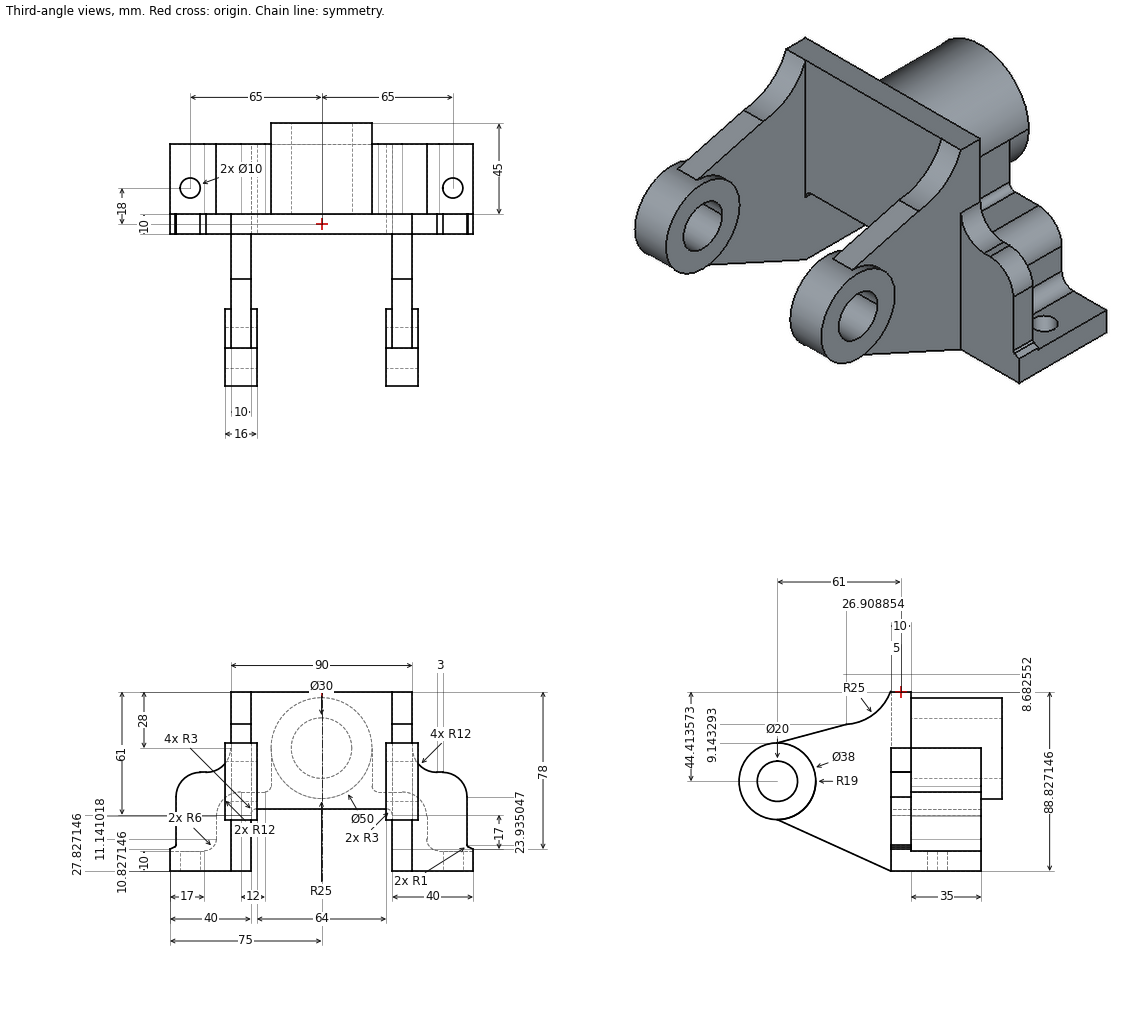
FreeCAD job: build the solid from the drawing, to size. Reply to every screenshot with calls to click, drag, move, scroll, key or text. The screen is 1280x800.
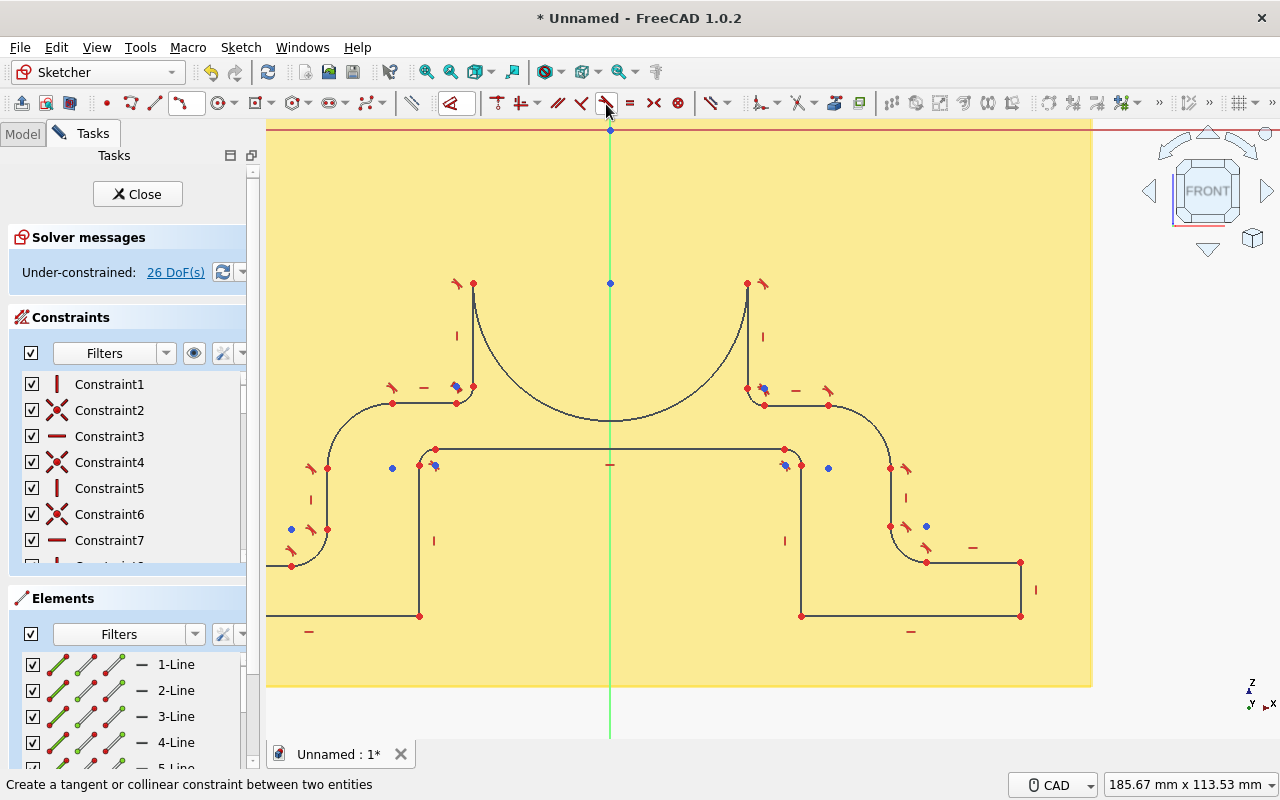
click(680, 449)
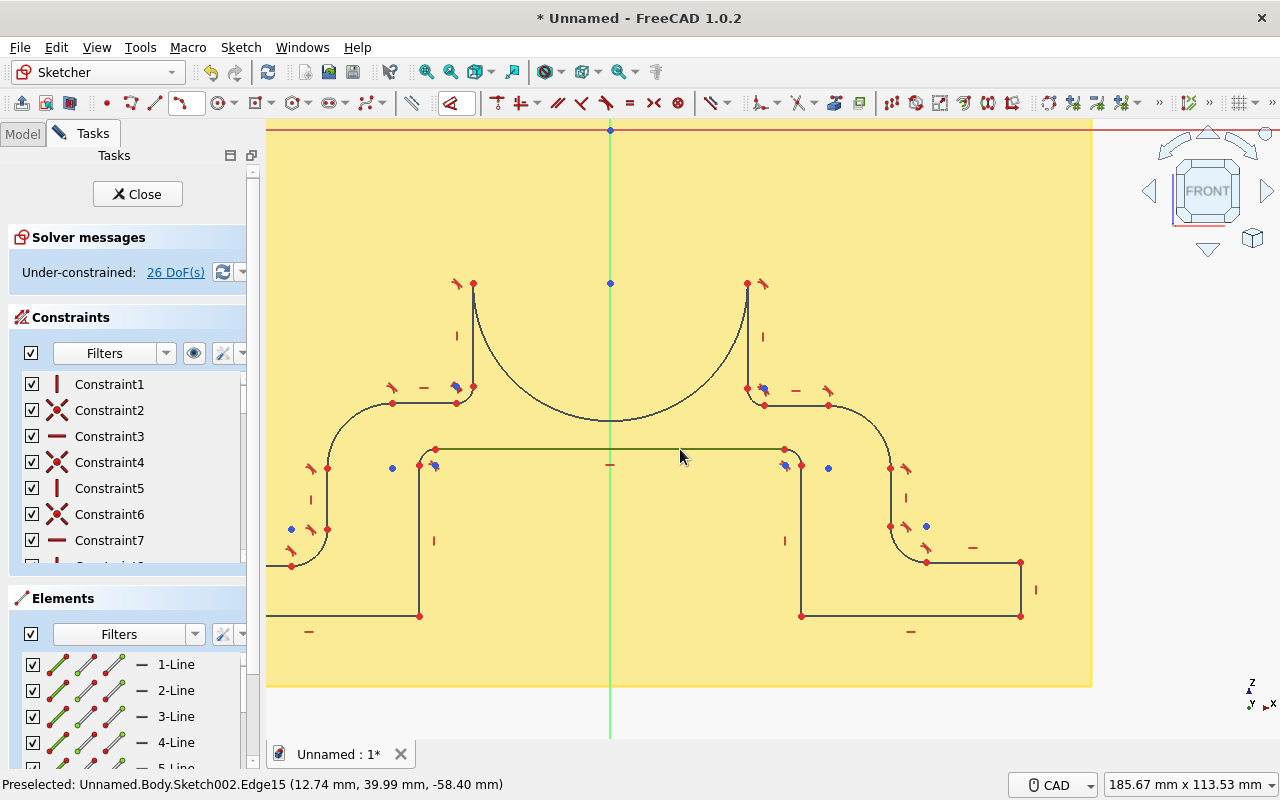
click(797, 454)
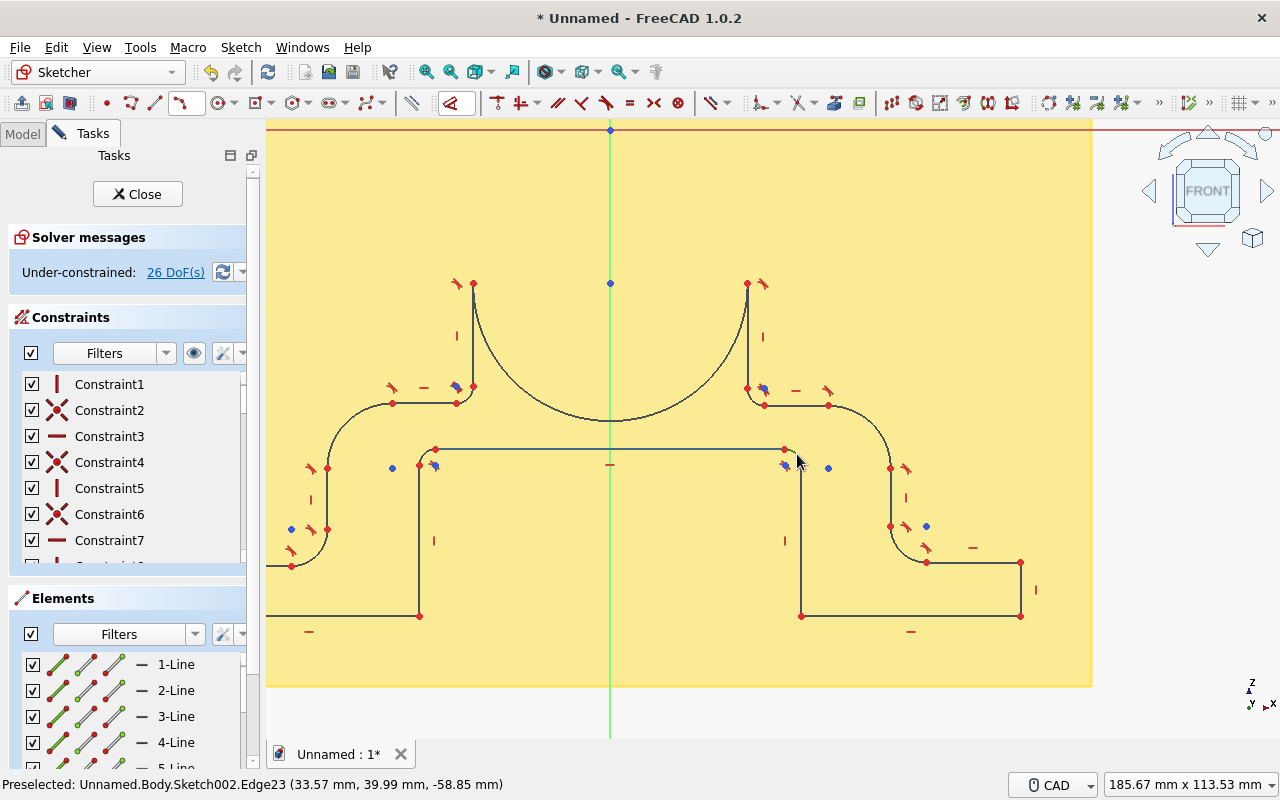
key(t)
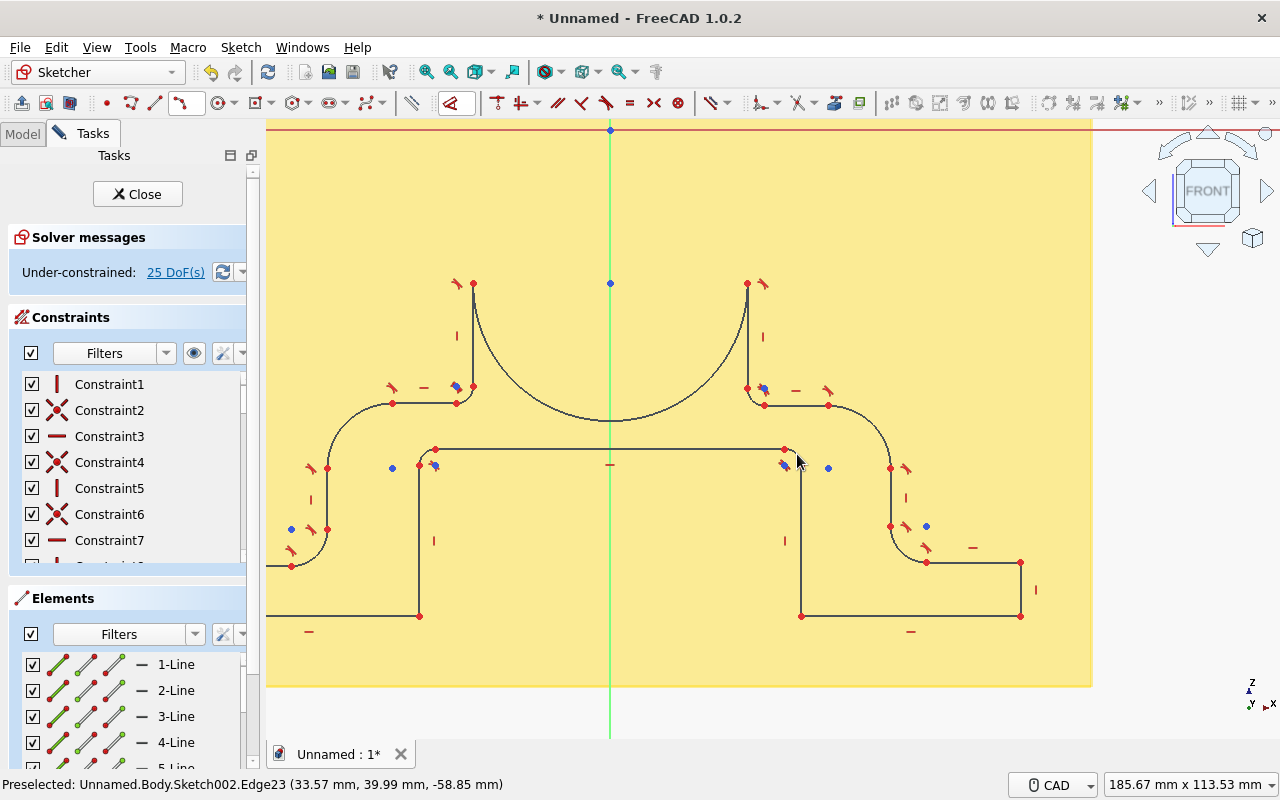
click(680, 449)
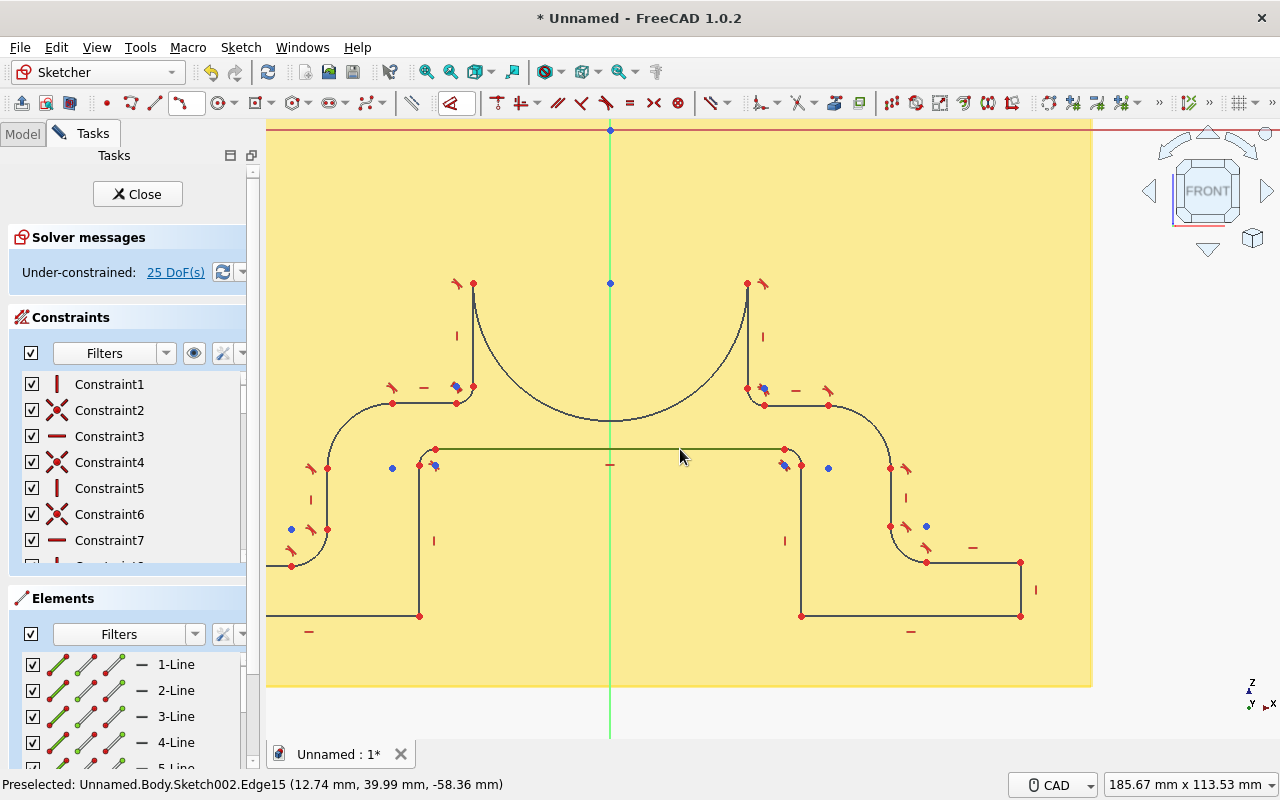
click(424, 454)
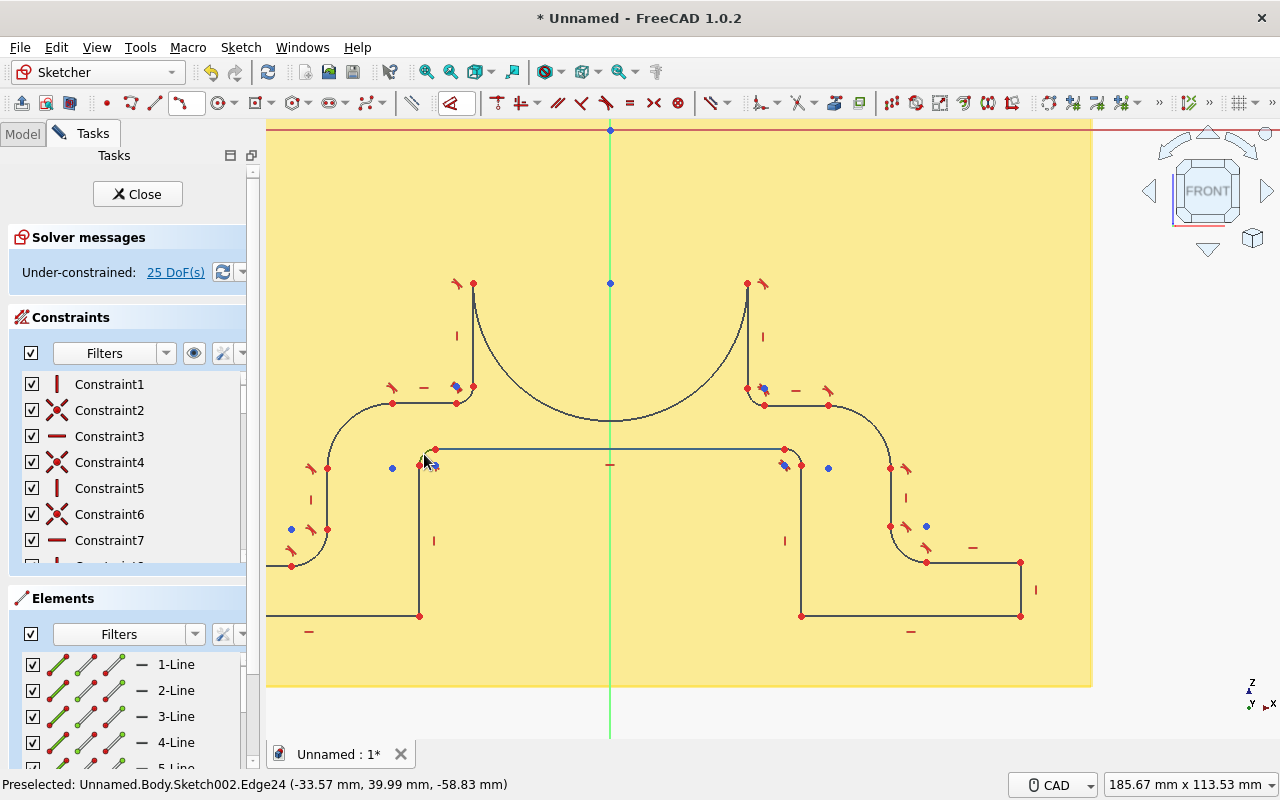
key(t)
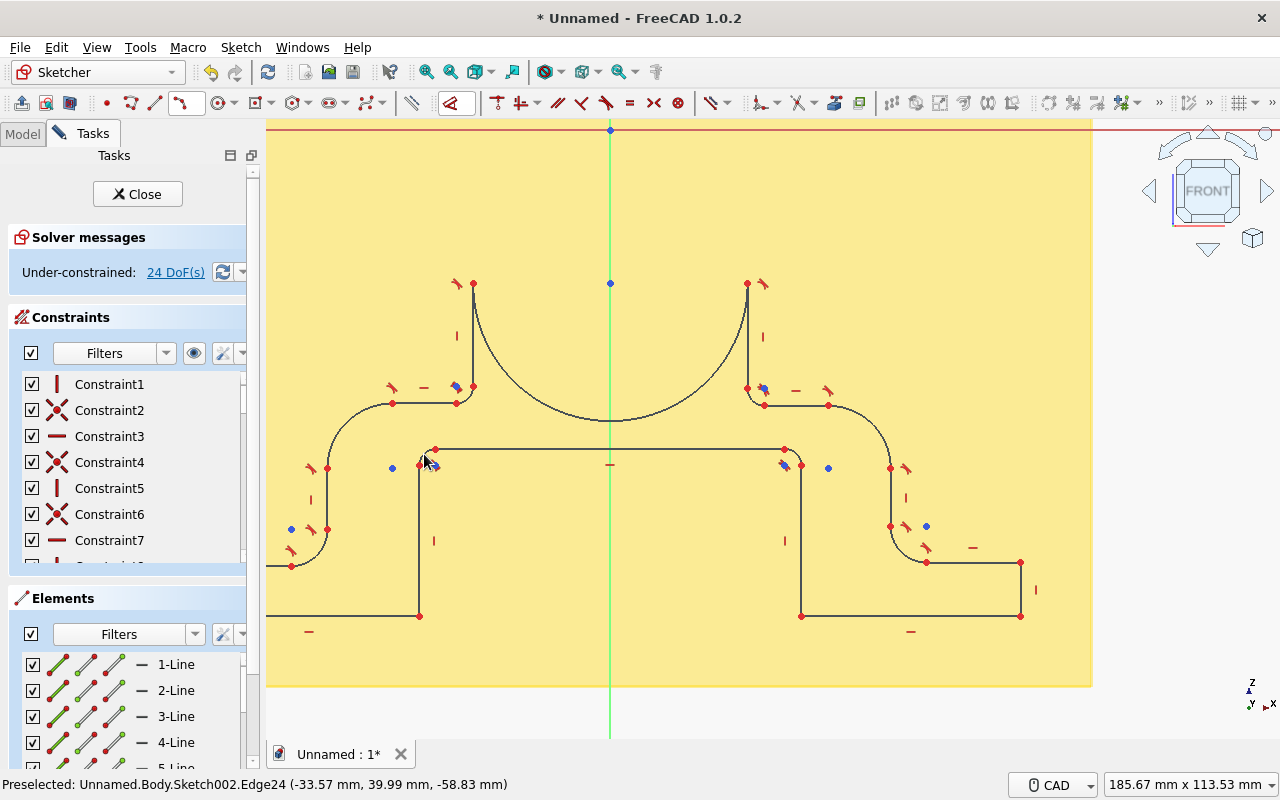
click(468, 399)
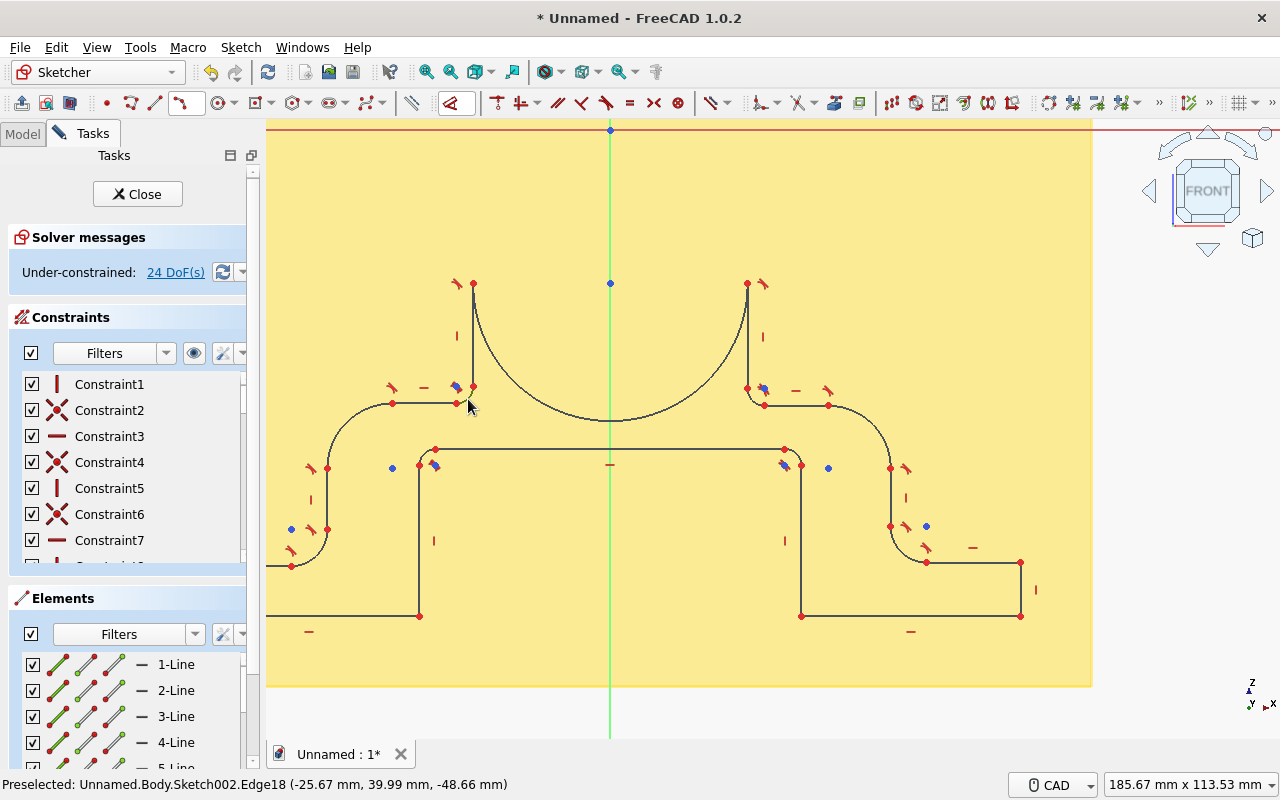
click(753, 401)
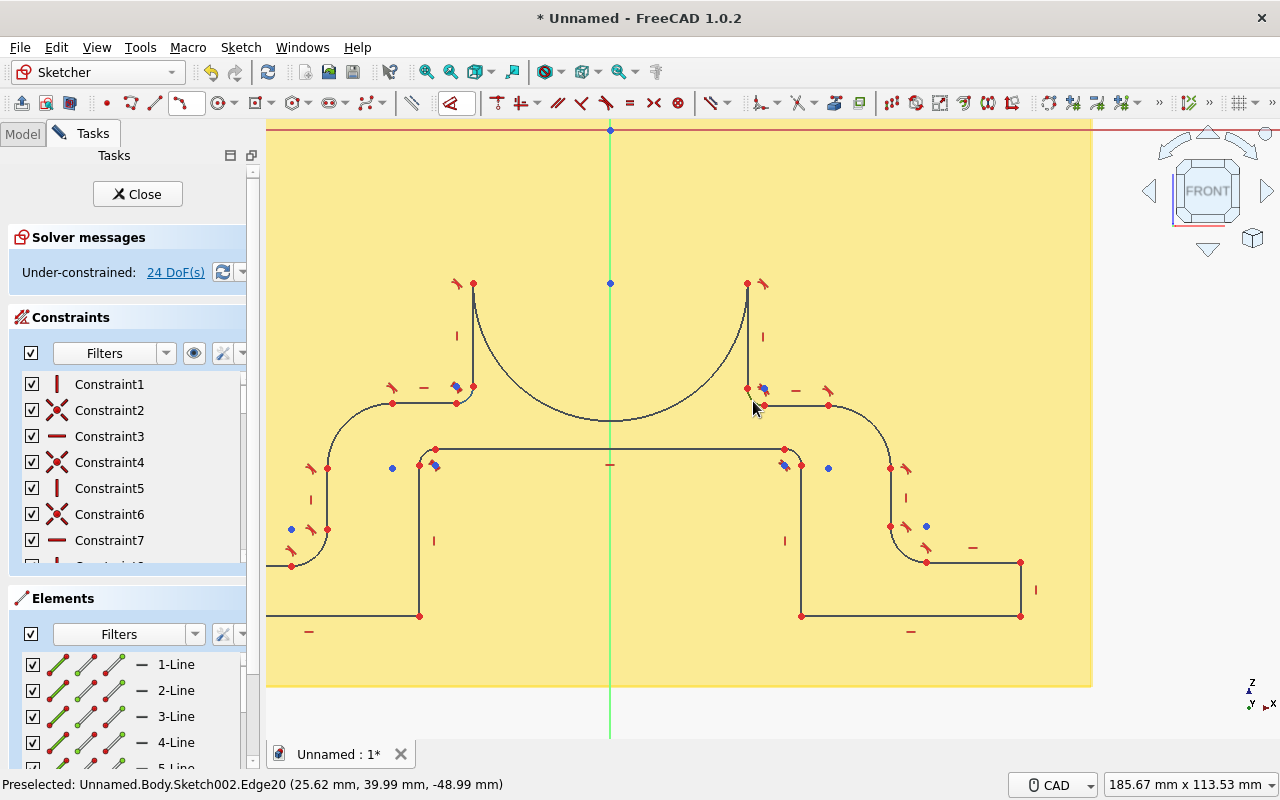
click(797, 454)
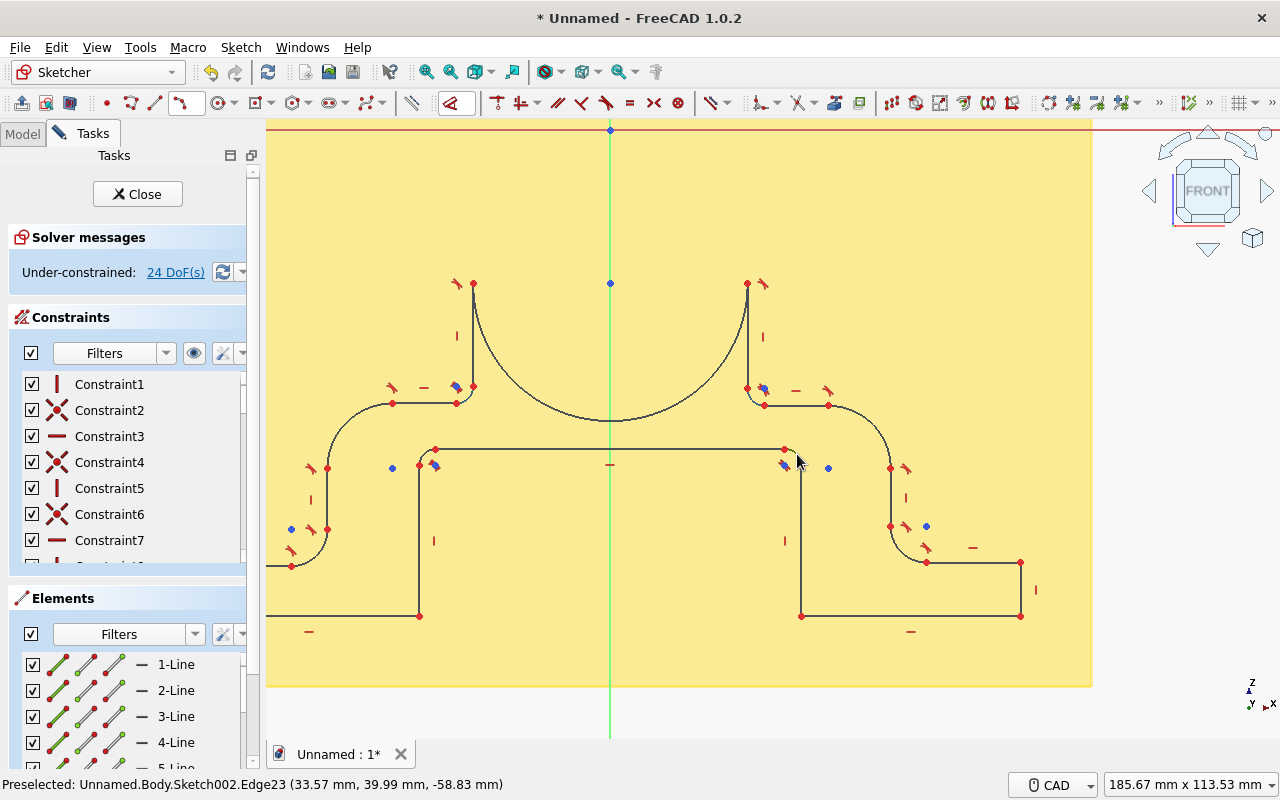
click(424, 454)